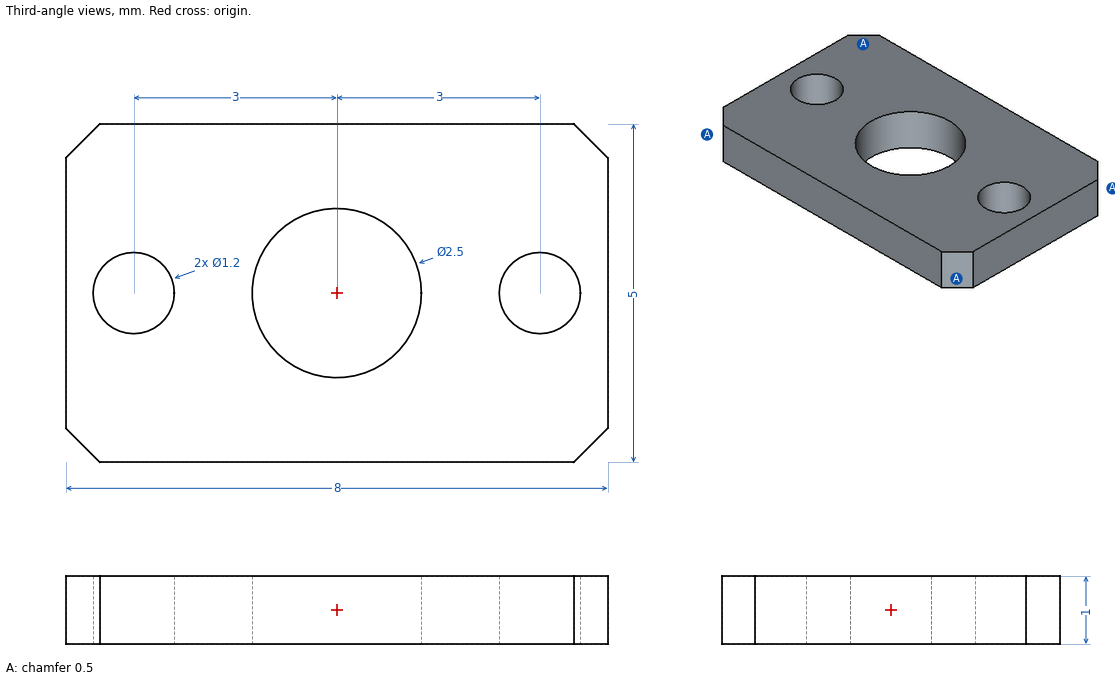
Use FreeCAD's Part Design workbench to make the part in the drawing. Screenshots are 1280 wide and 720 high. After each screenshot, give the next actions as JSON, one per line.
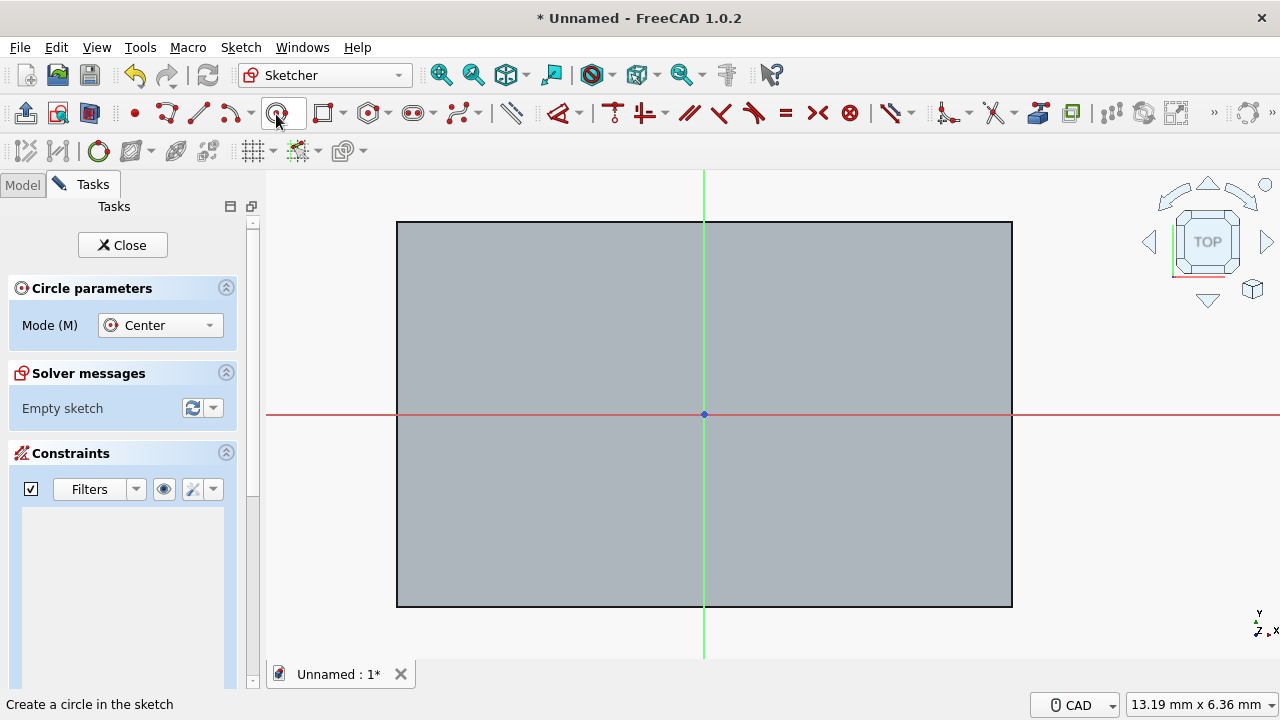
{"action": "left_click", "coordinate": [704, 414]}
{"action": "left_click", "coordinate": [772, 347]}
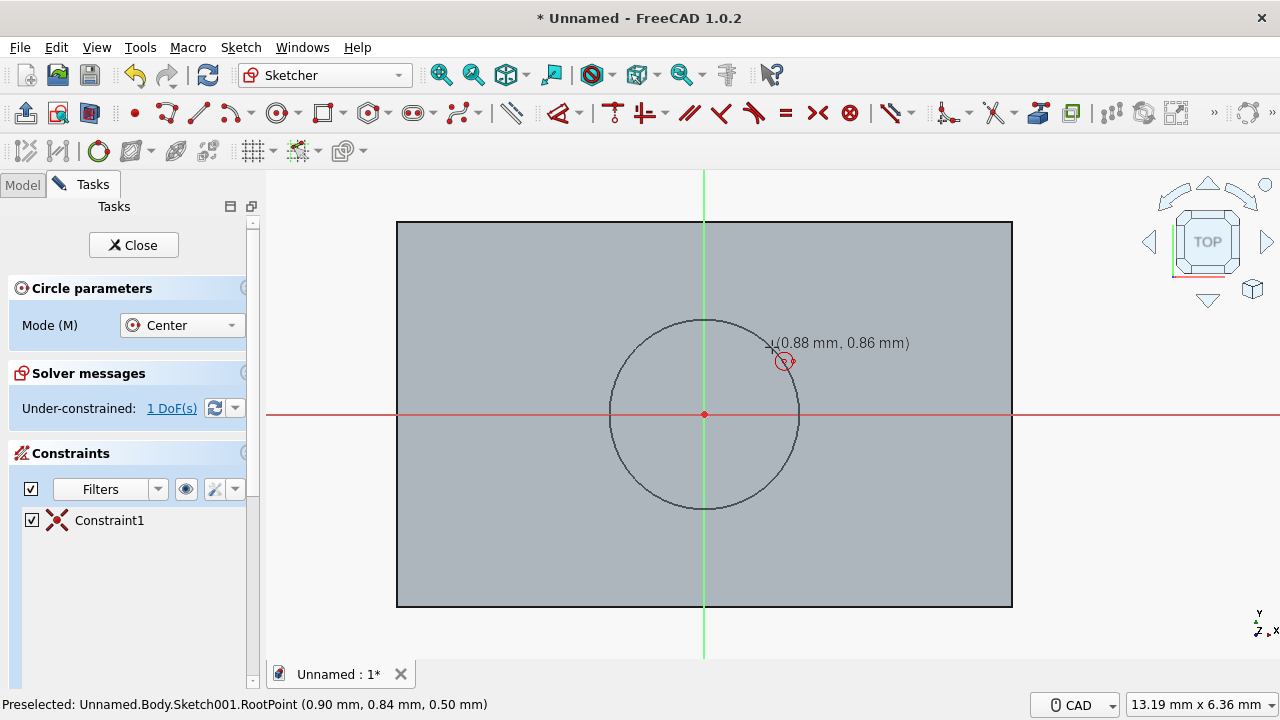
{"action": "left_click", "coordinate": [474, 414]}
{"action": "left_click", "coordinate": [506, 382]}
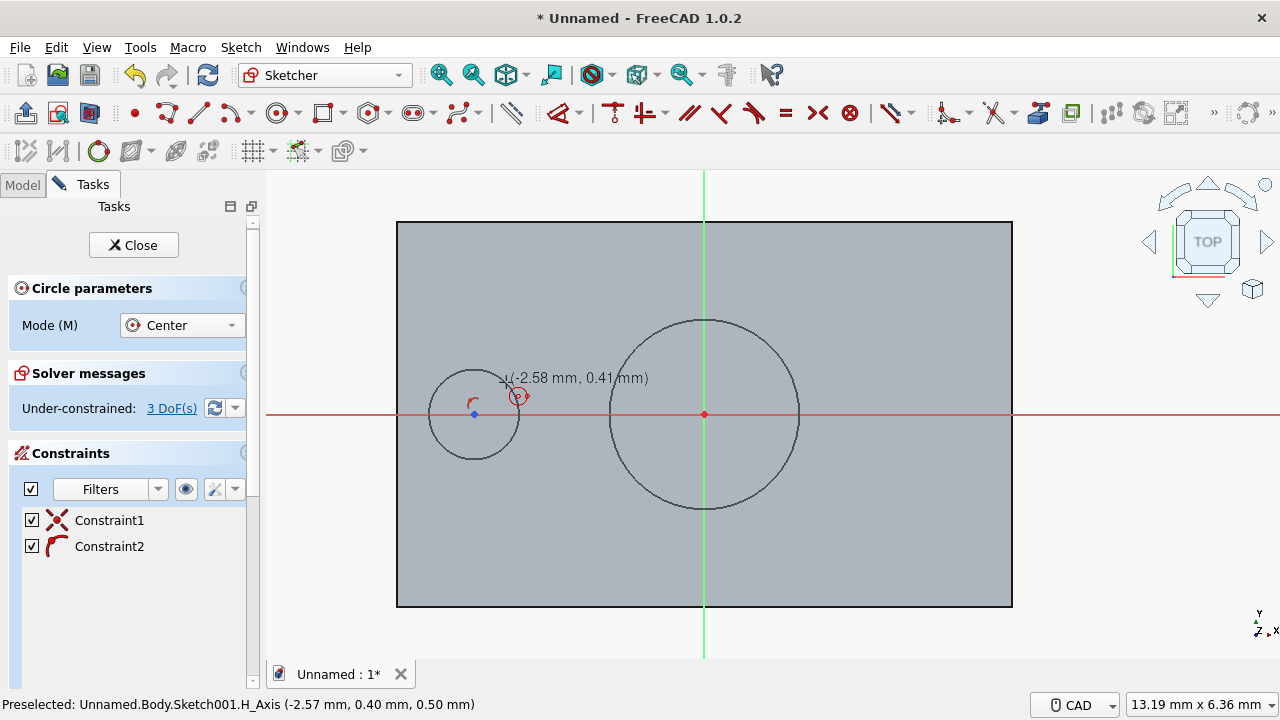
{"action": "left_click", "coordinate": [935, 414]}
{"action": "left_click", "coordinate": [968, 382]}
{"action": "key", "text": "Escape"}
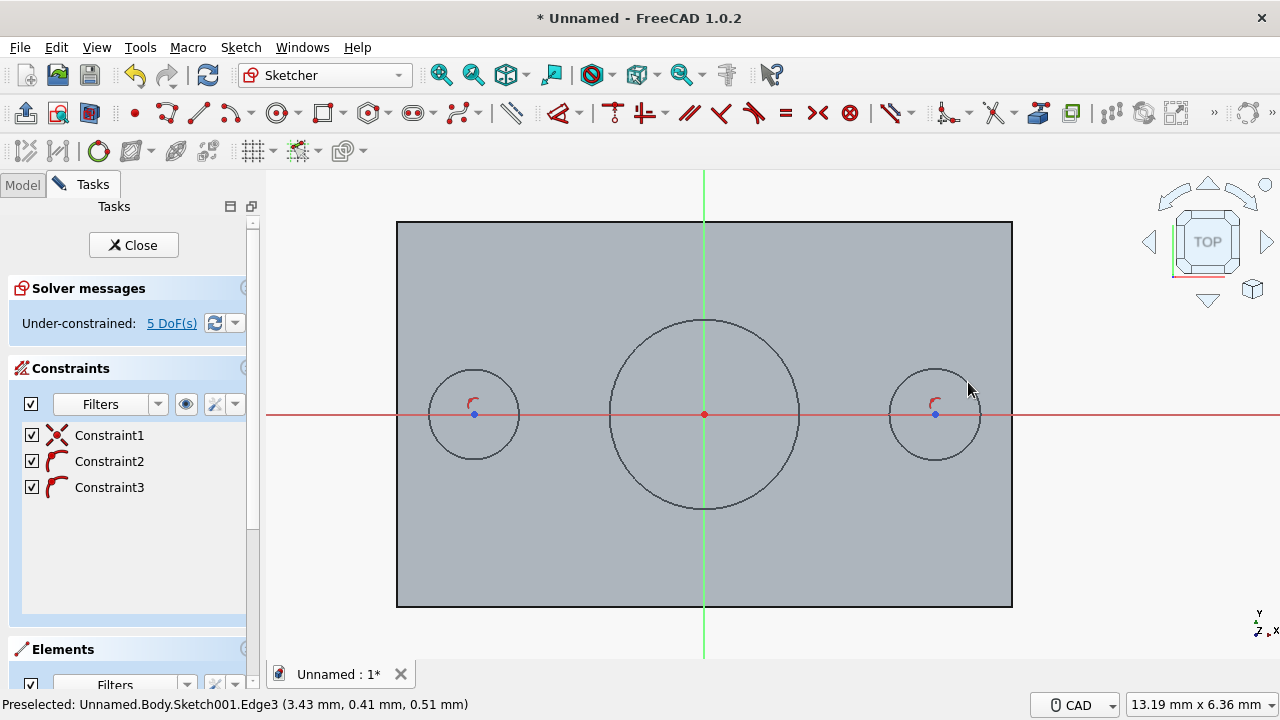
{"action": "left_click", "coordinate": [506, 383]}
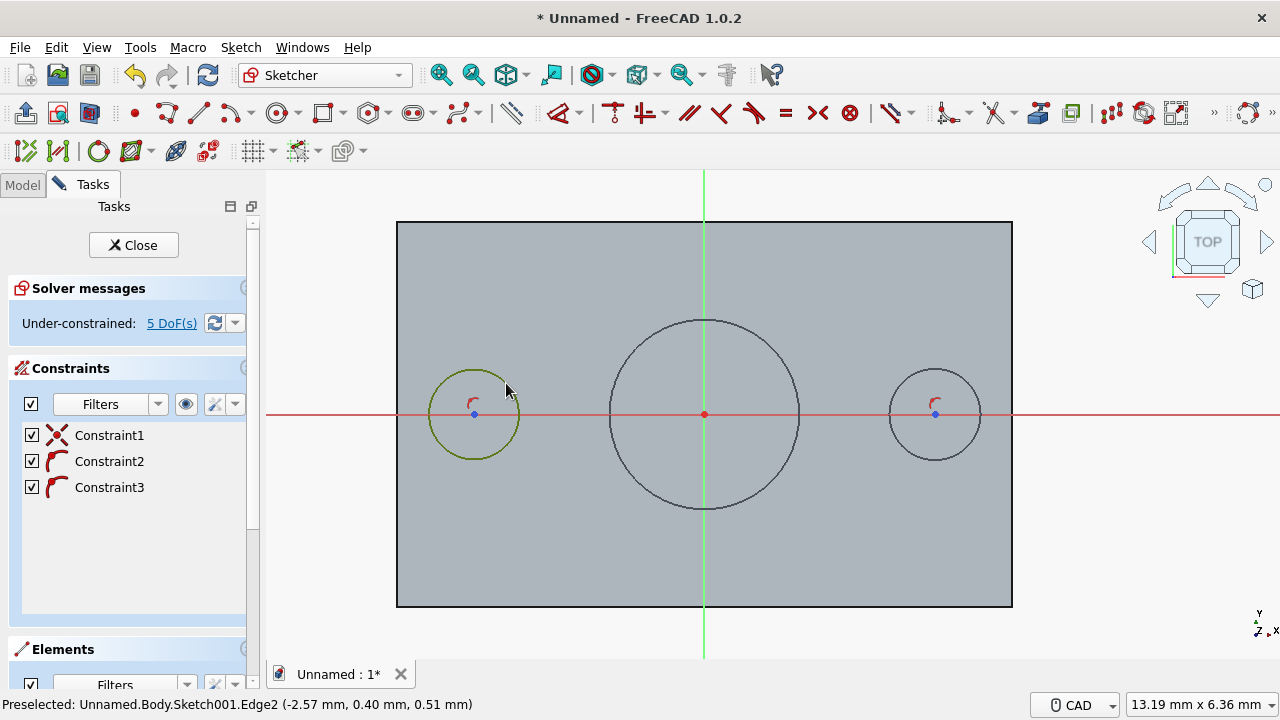
{"action": "left_click", "coordinate": [967, 382]}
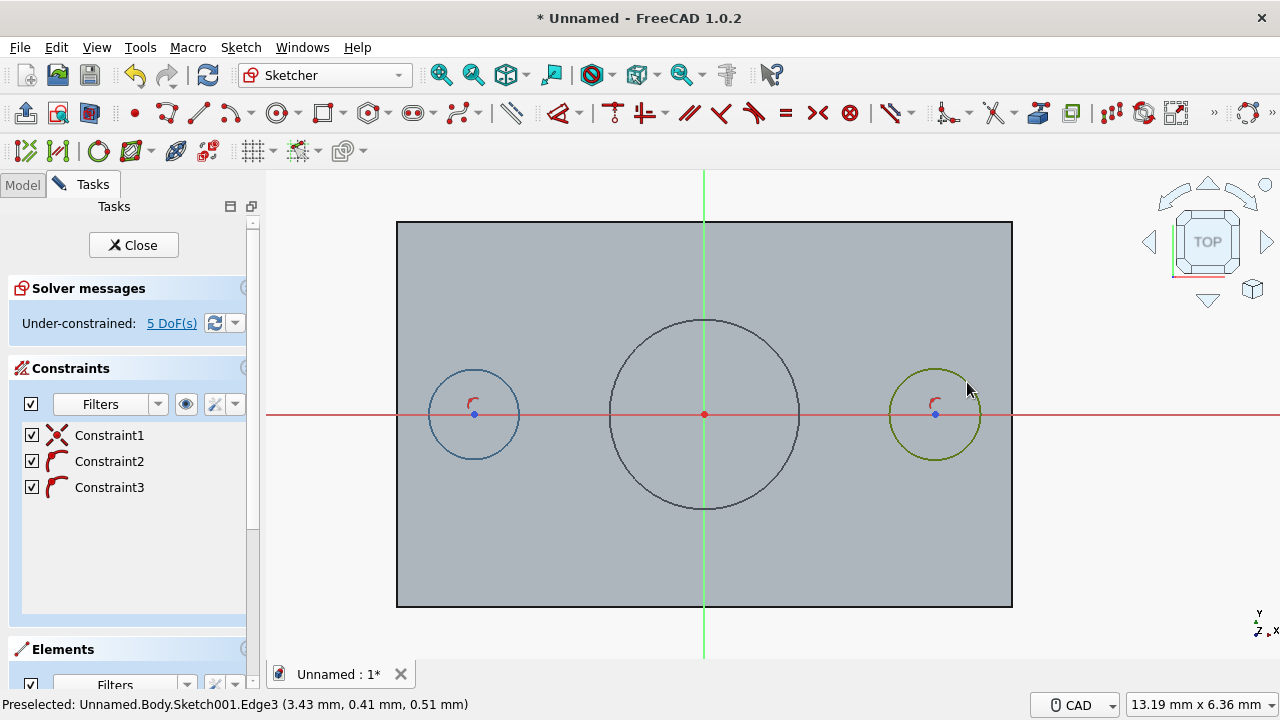
{"action": "left_click", "coordinate": [786, 114]}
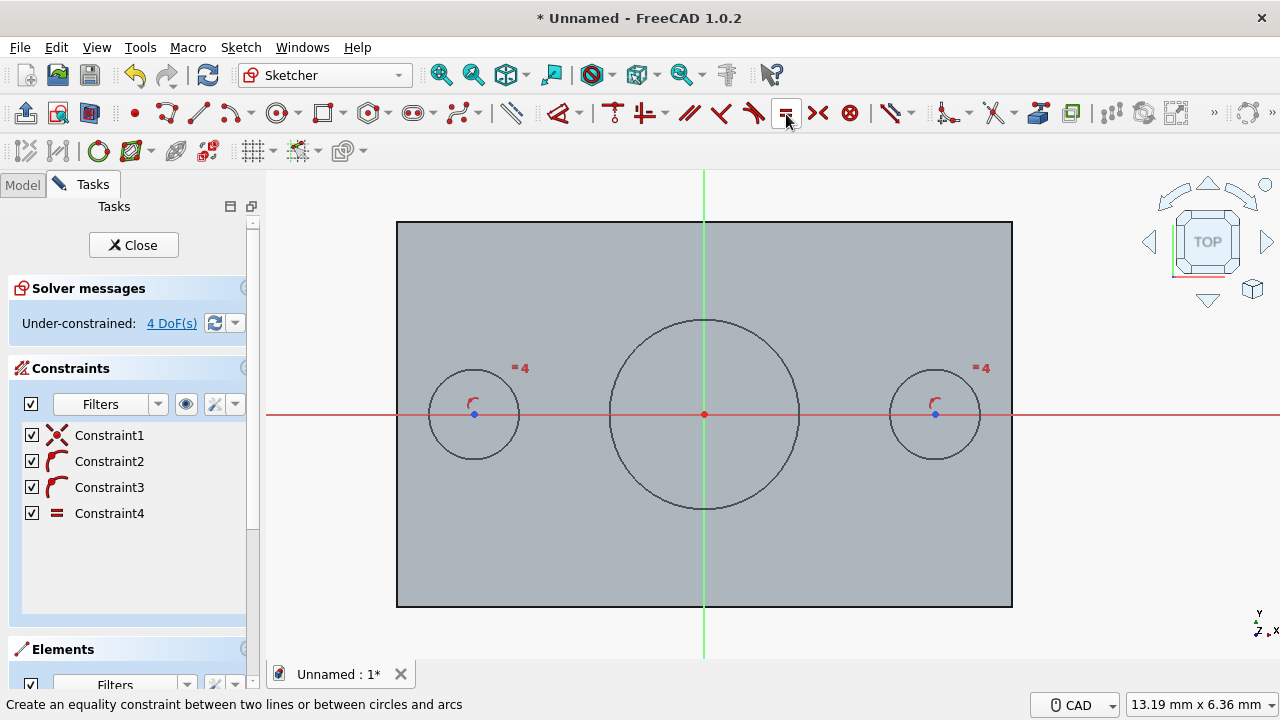
{"action": "left_click", "coordinate": [558, 114]}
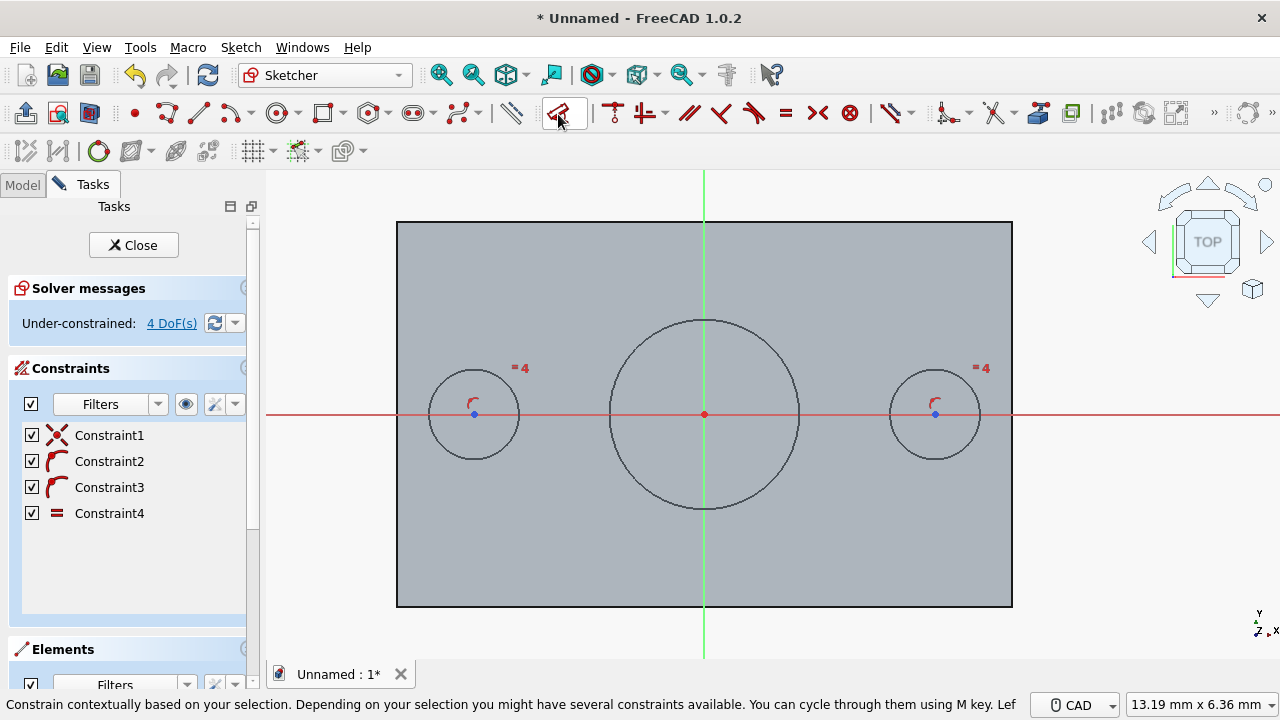
{"action": "left_click", "coordinate": [771, 347]}
{"action": "left_click", "coordinate": [793, 324]}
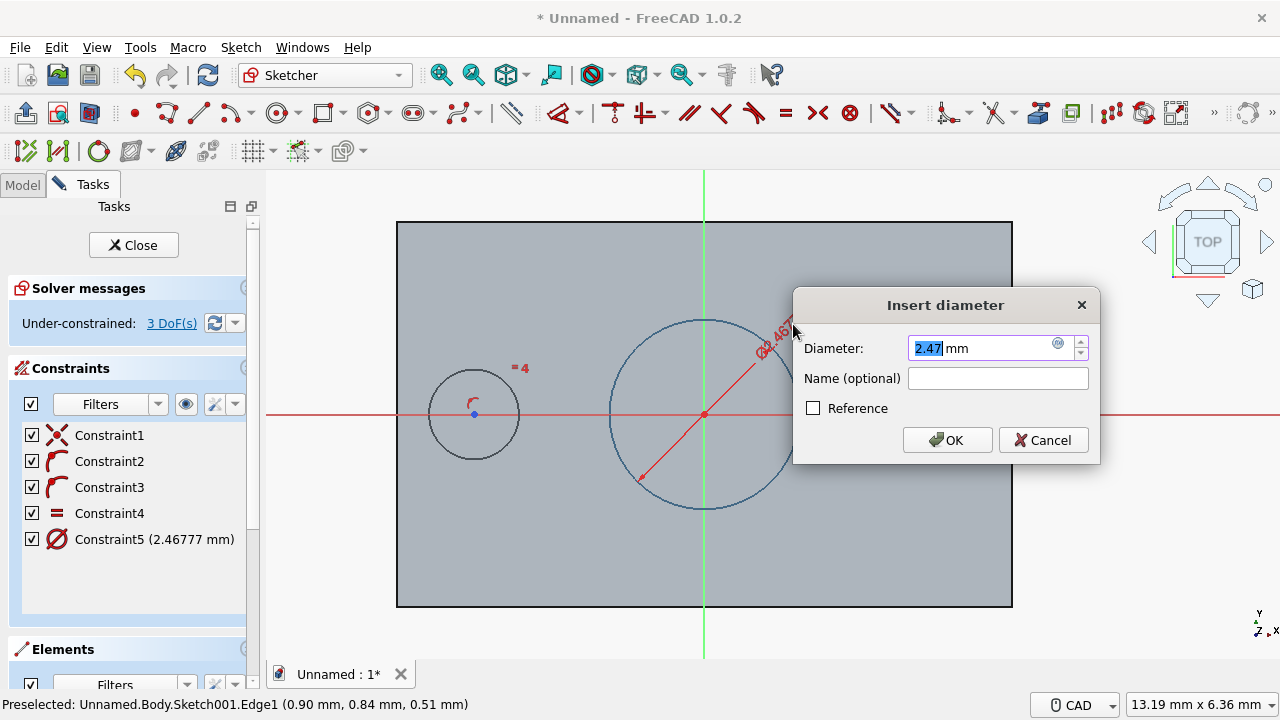
{"action": "type", "text": "2.5"}
{"action": "key", "text": "Return"}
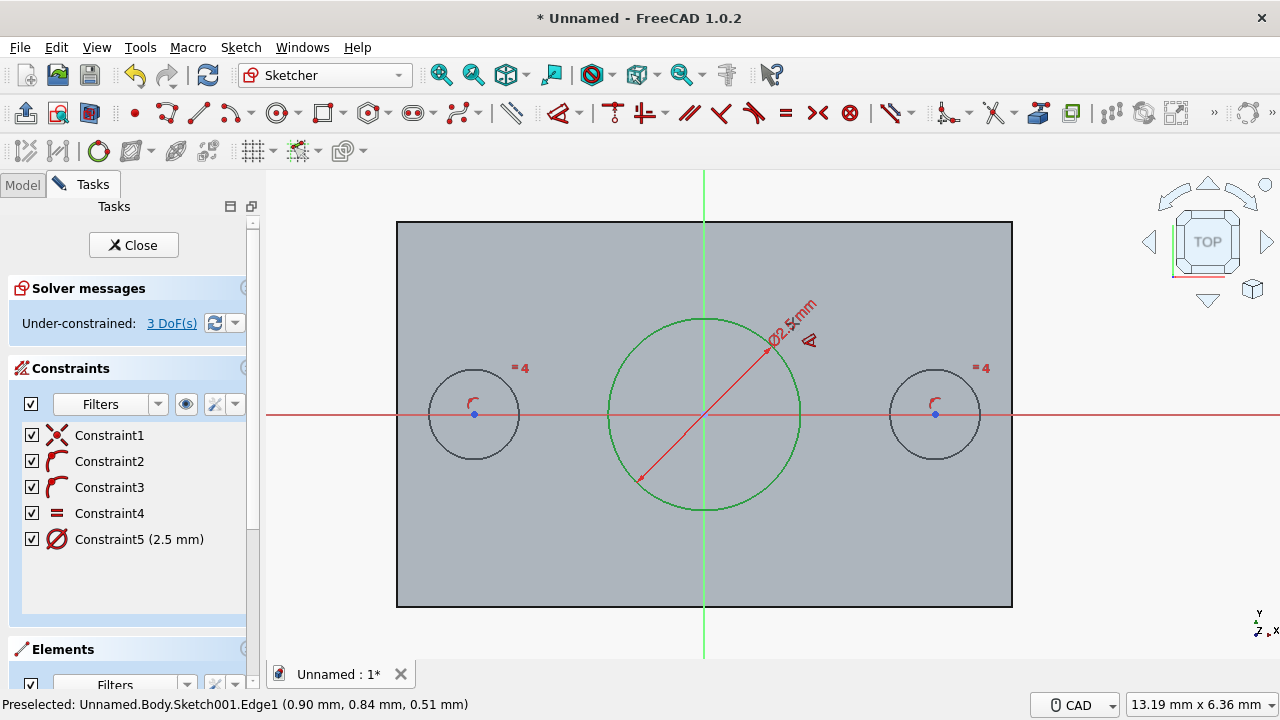
{"action": "left_click", "coordinate": [506, 383]}
{"action": "left_click", "coordinate": [529, 361]}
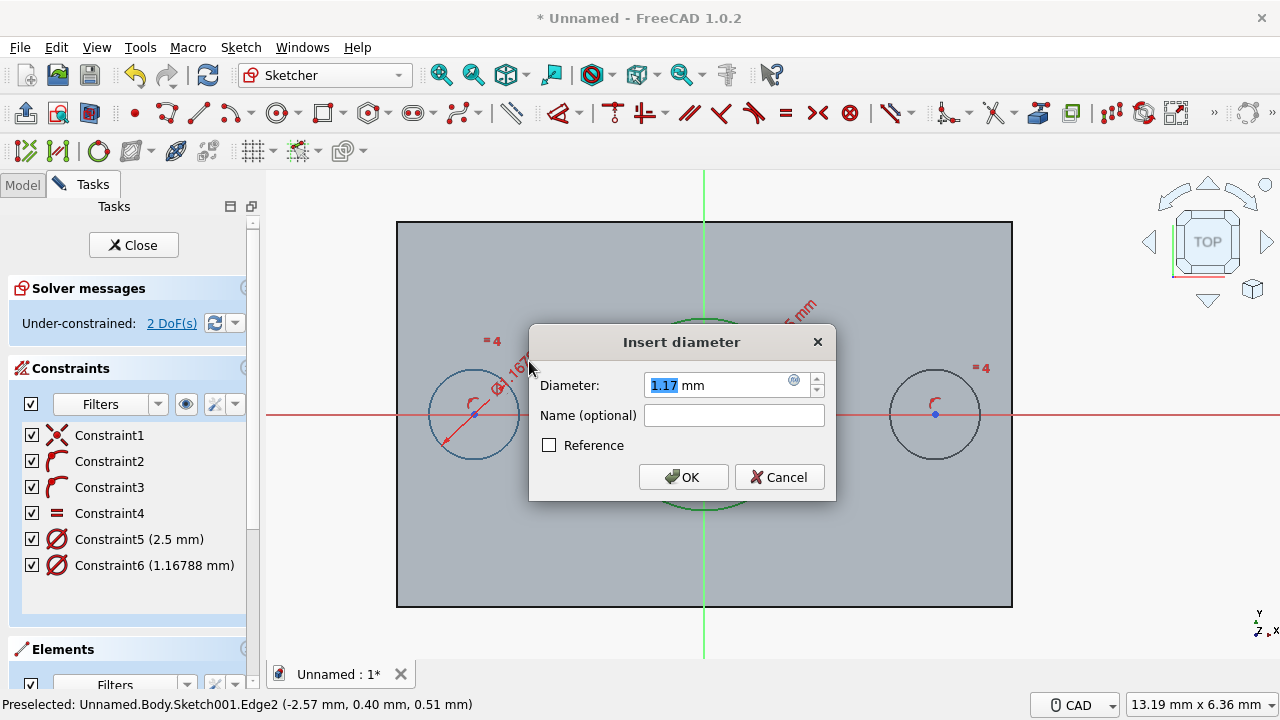
{"action": "type", "text": "1.2"}
{"action": "key", "text": "Return"}